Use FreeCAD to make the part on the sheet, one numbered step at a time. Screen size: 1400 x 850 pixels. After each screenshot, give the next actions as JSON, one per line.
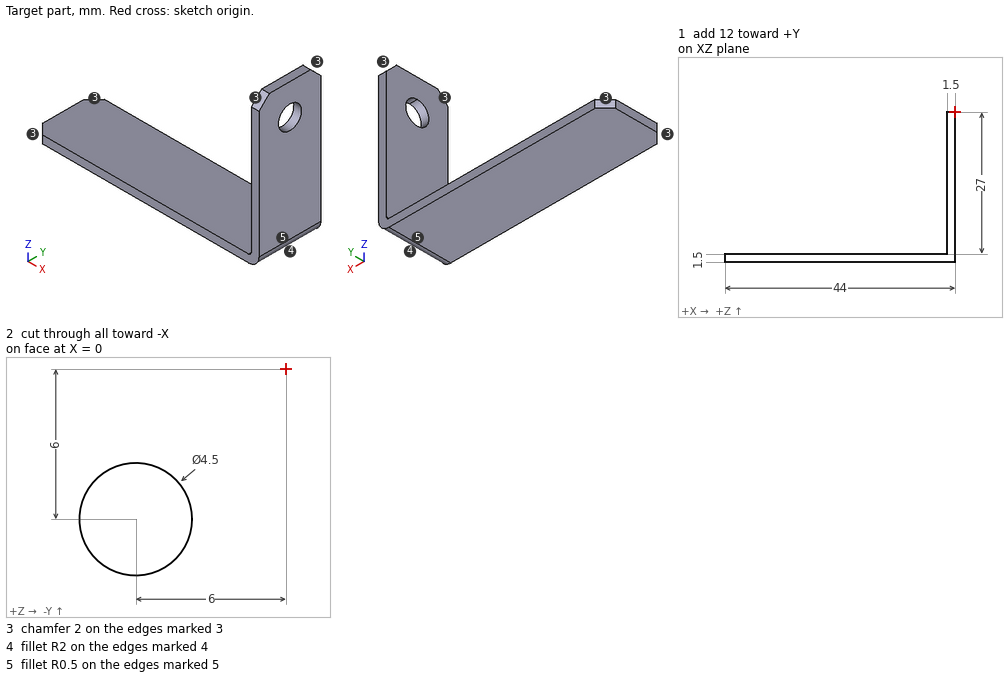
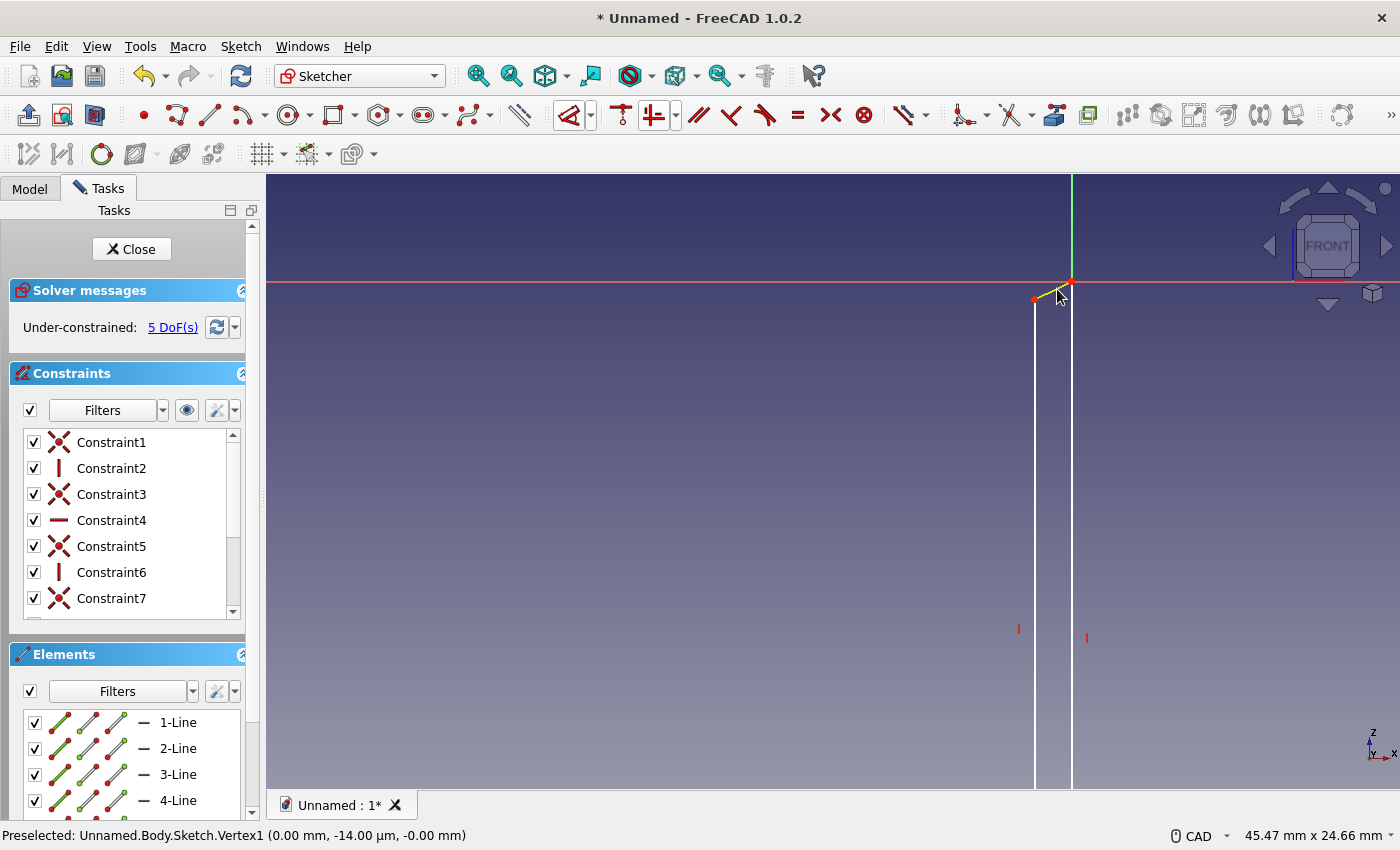
{"action": "left_click", "coordinate": [1057, 289]}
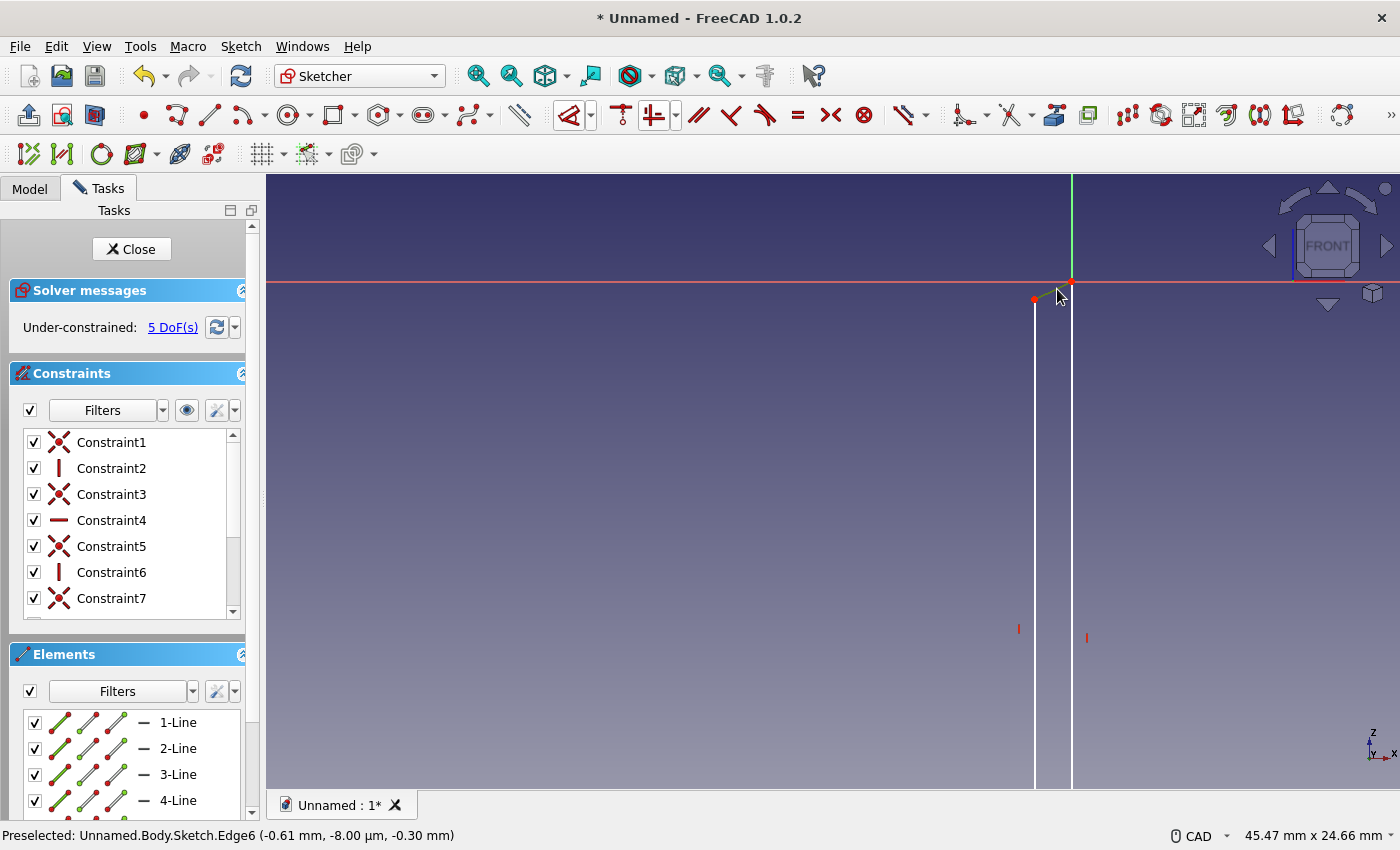
{"action": "key", "text": "h"}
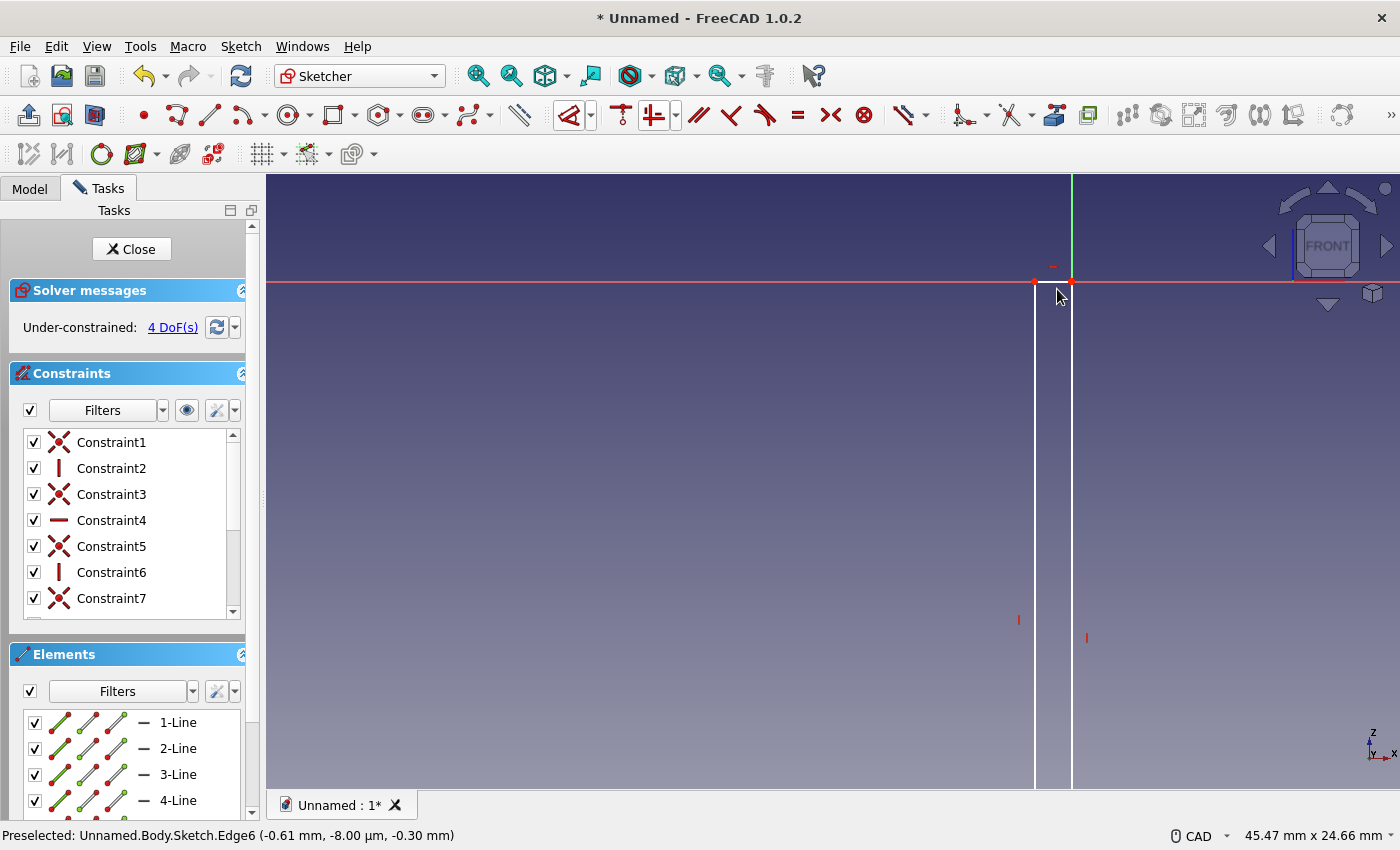
{"action": "scroll", "coordinate": [1058, 292], "scroll_direction": "down", "scroll_amount": 3}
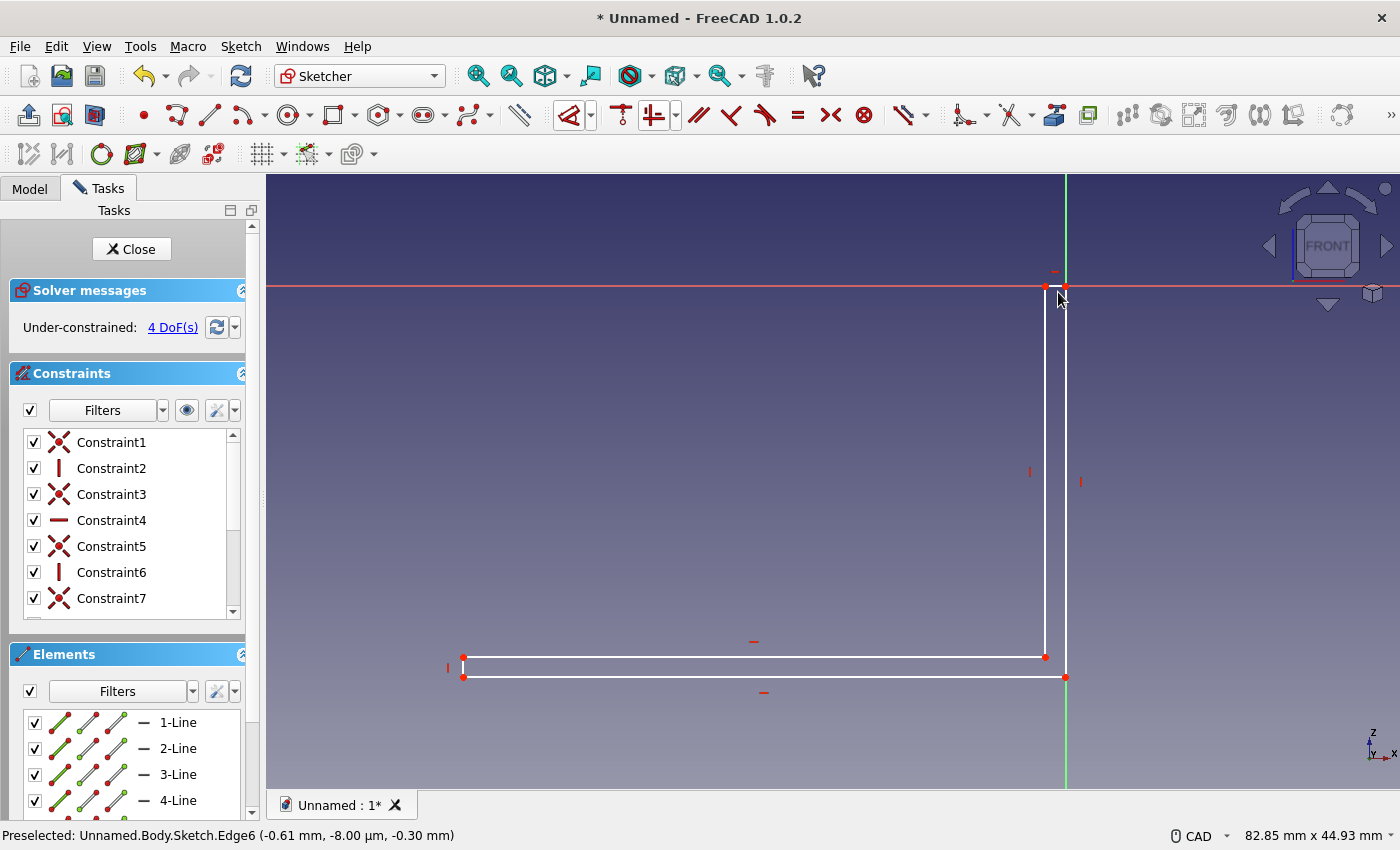
{"action": "left_click", "coordinate": [885, 677]}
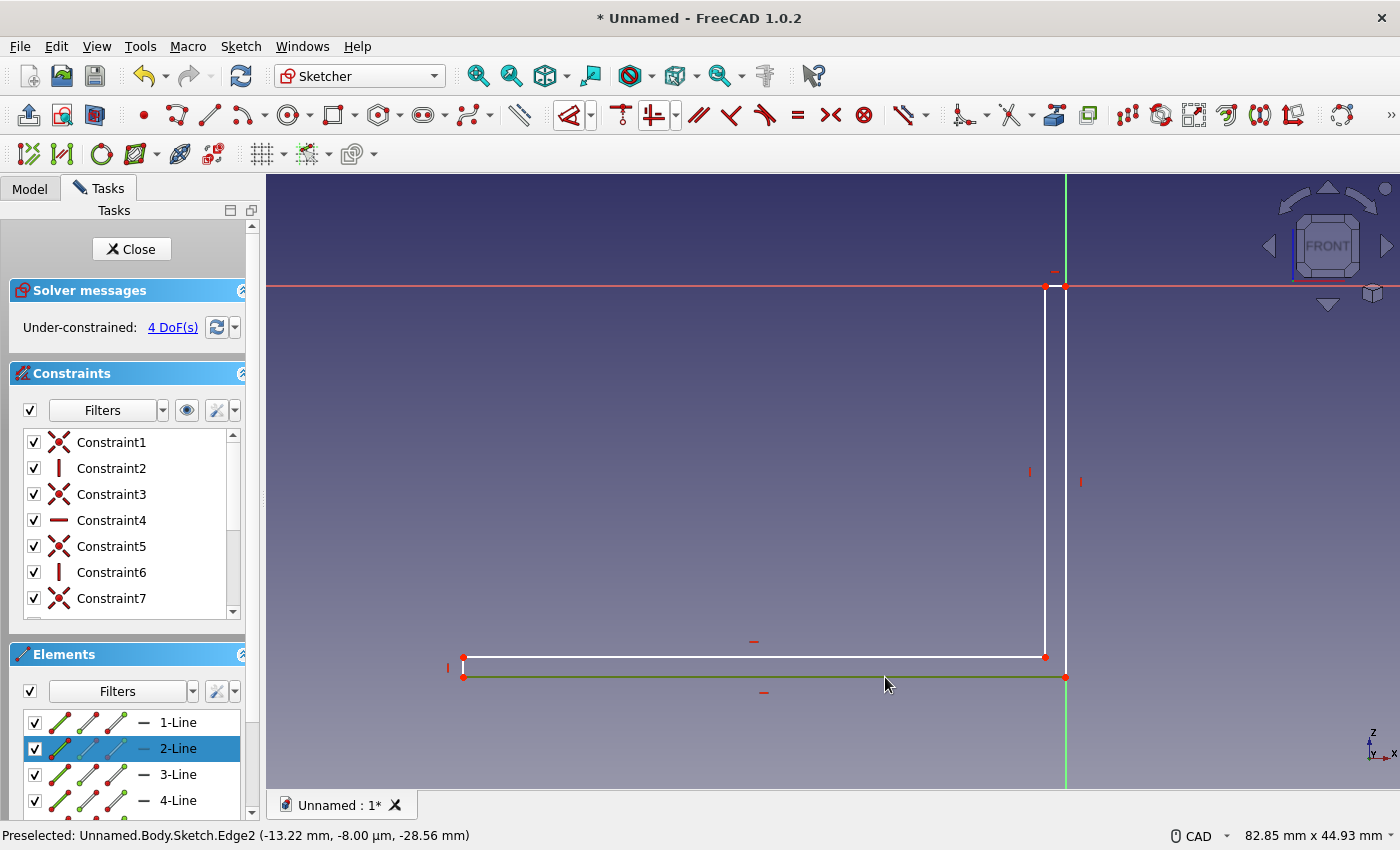
{"action": "key", "text": "l"}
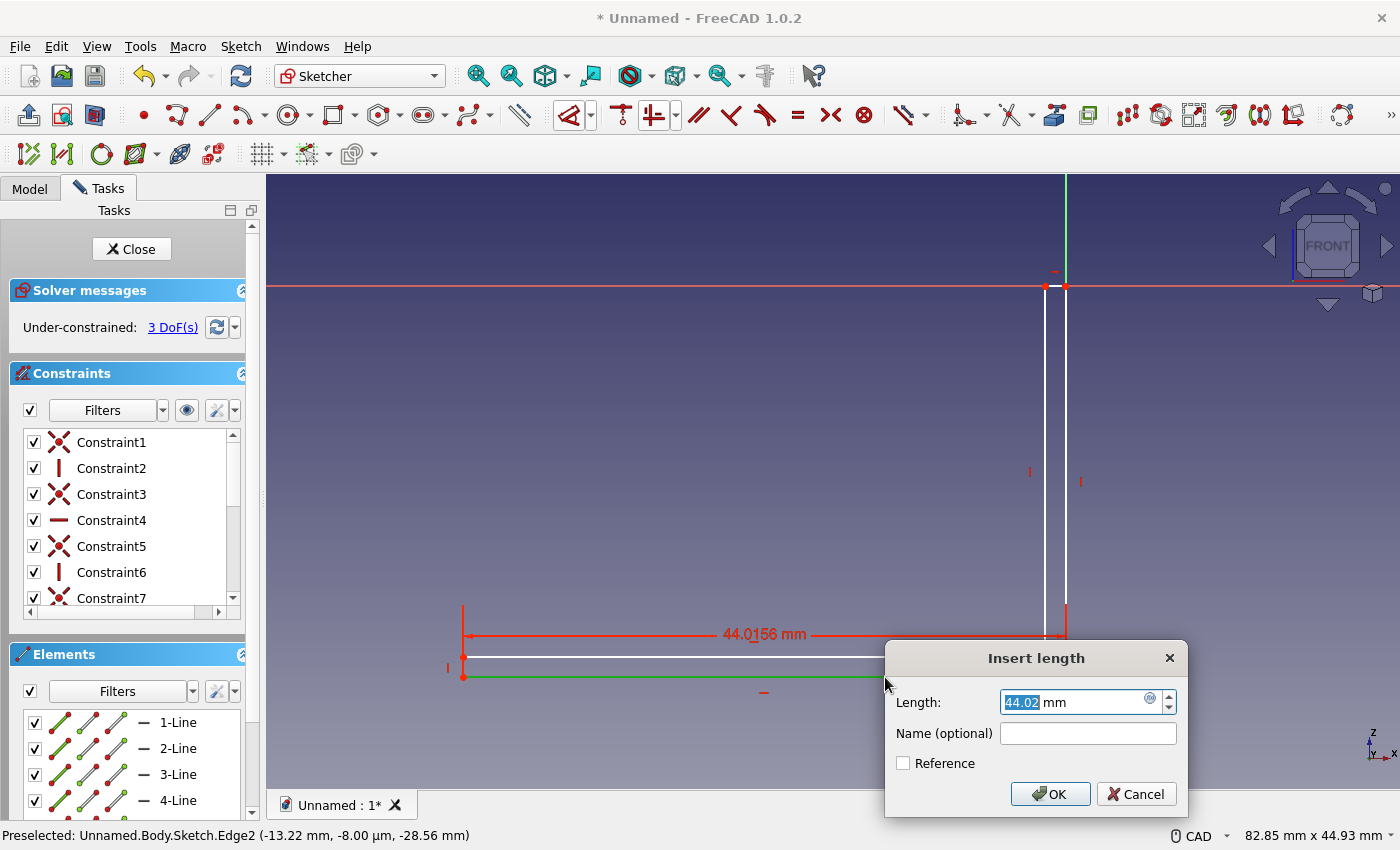
{"action": "type", "text": "44"}
{"action": "key", "text": "Return"}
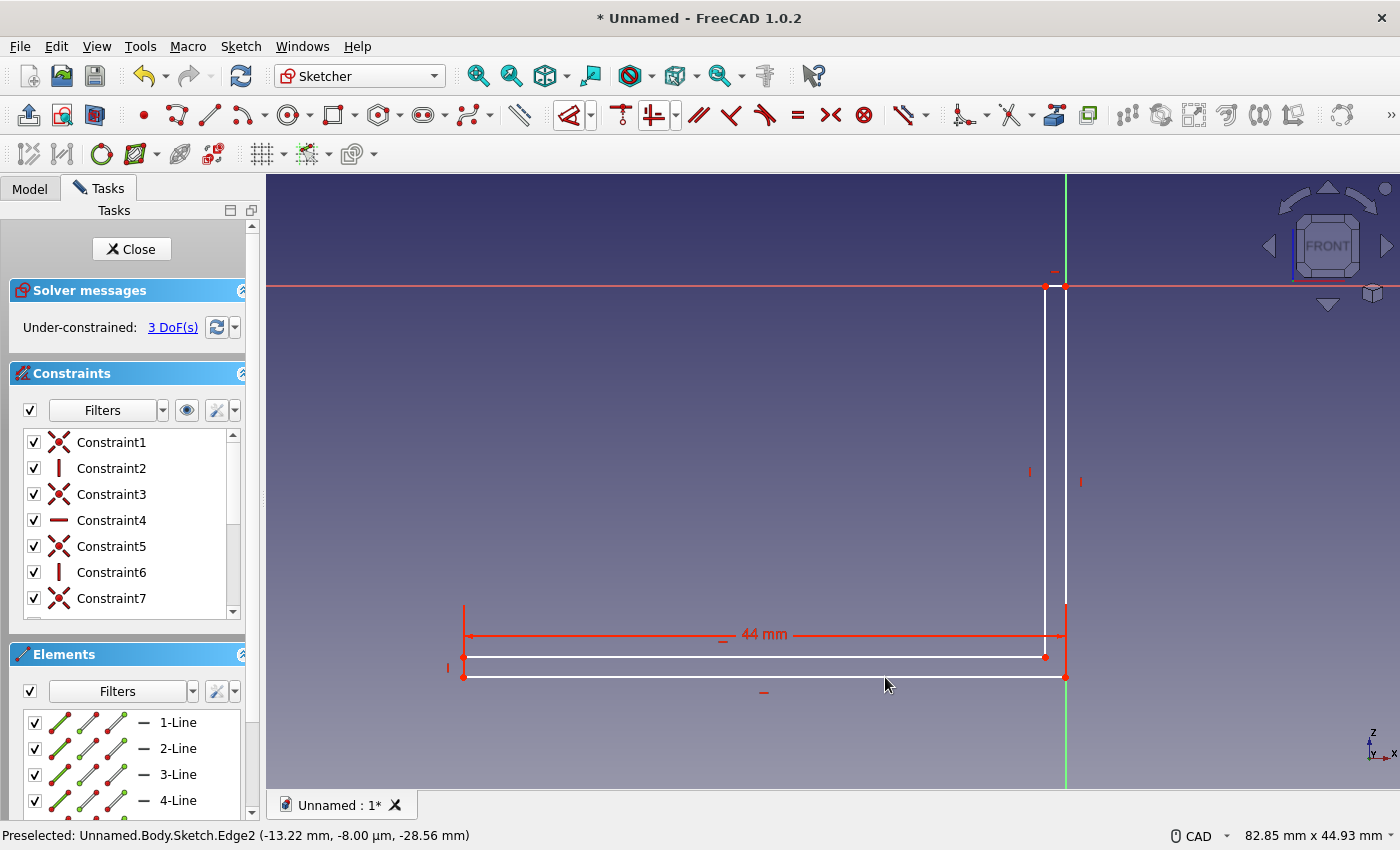
{"action": "left_click", "coordinate": [1045, 546]}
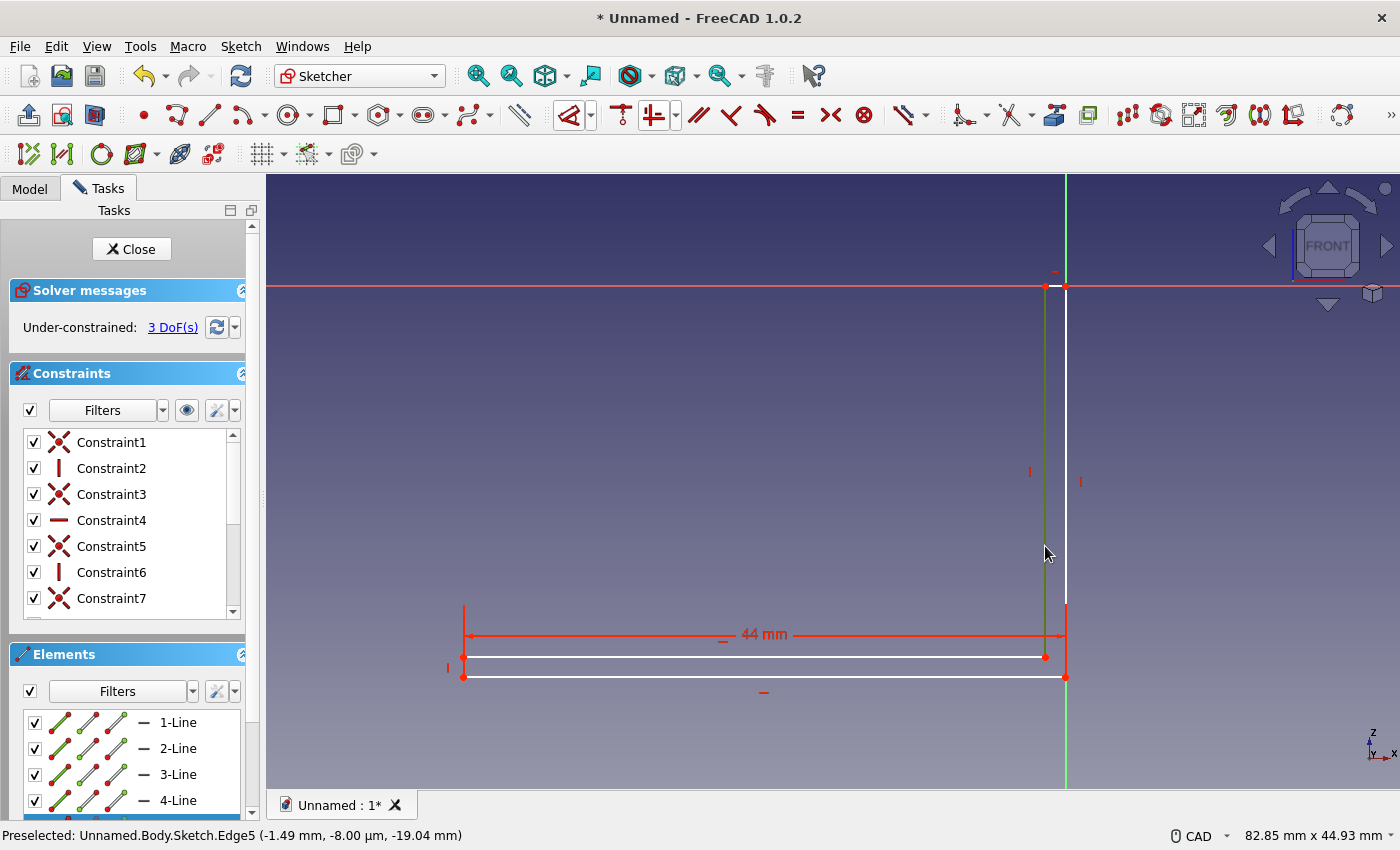
{"action": "key", "text": "i"}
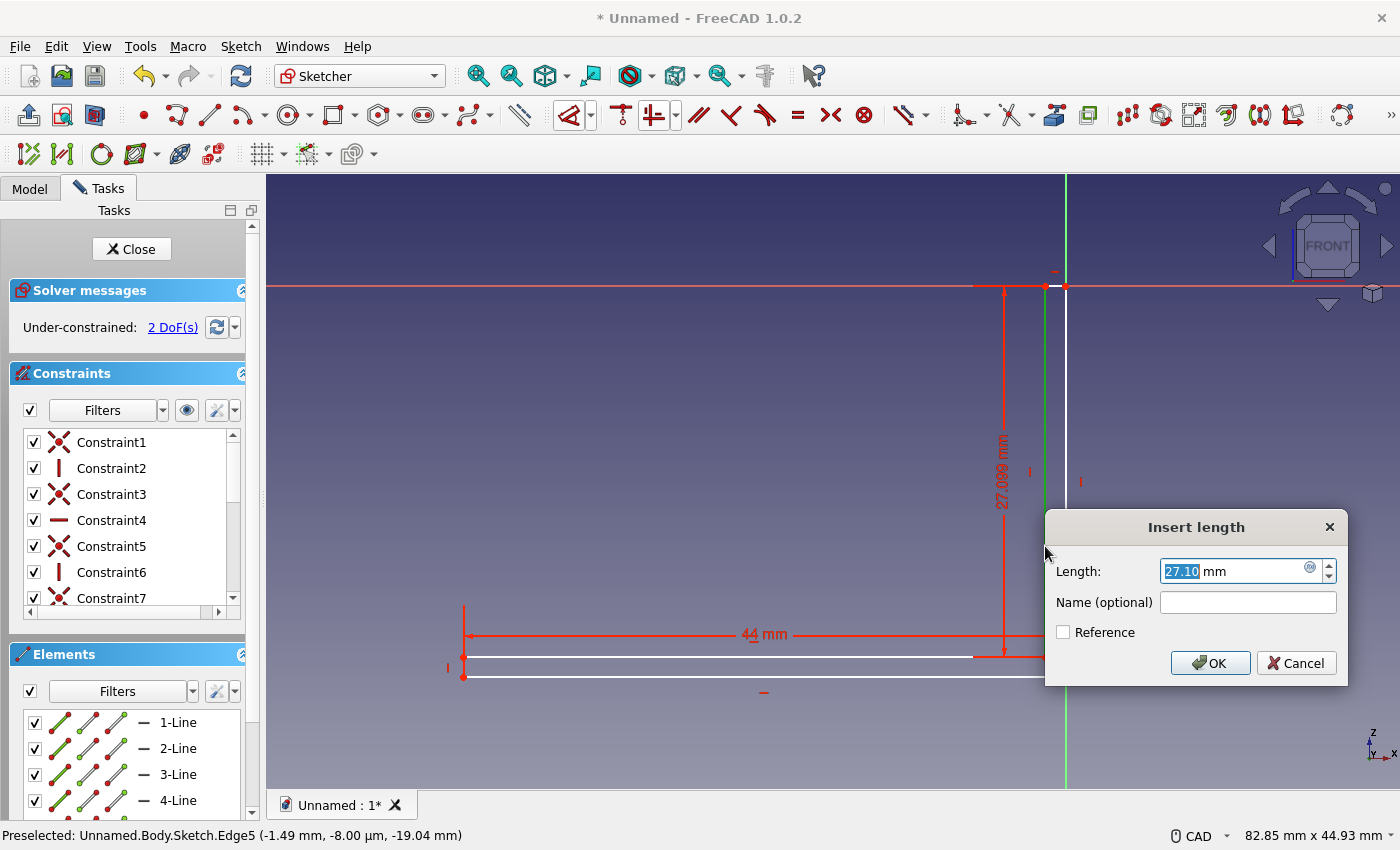
{"action": "type", "text": "27"}
{"action": "key", "text": "Return"}